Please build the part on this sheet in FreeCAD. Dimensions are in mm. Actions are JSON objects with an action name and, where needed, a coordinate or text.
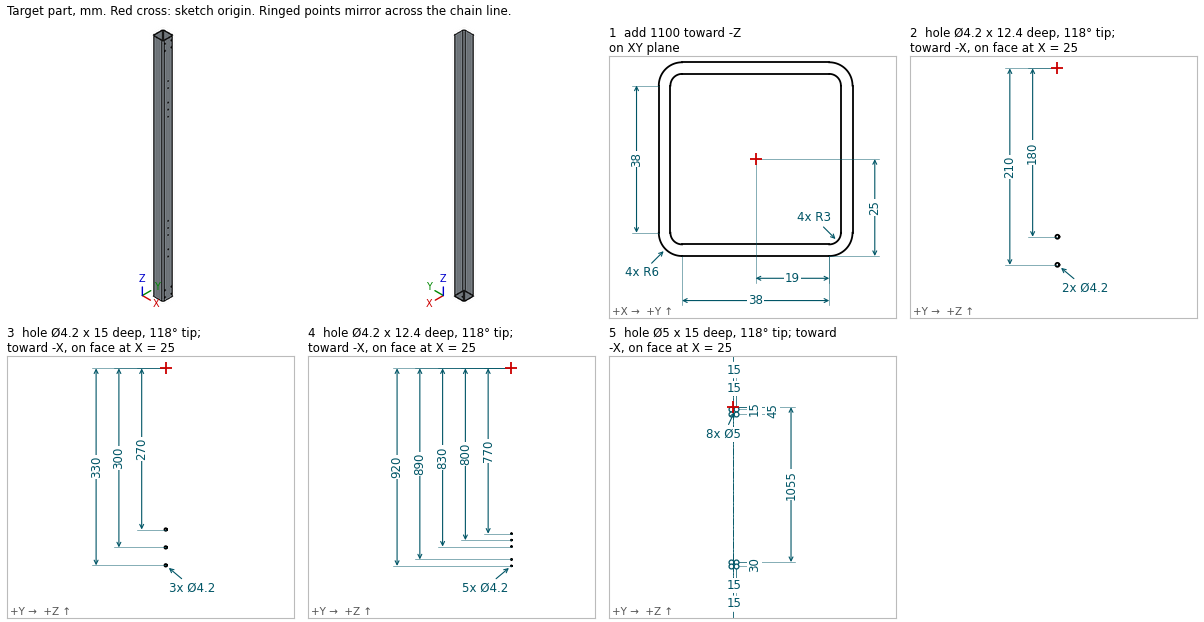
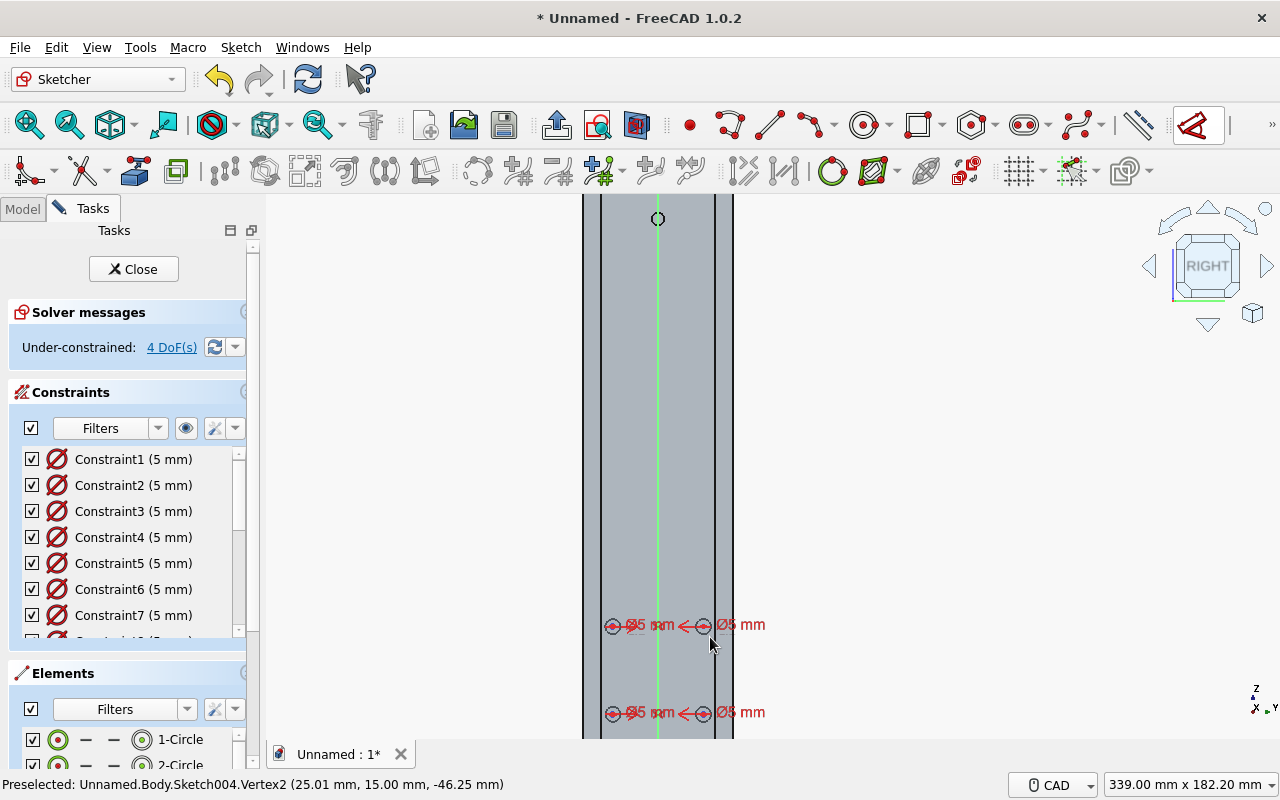
{"action": "left_click", "coordinate": [704, 627]}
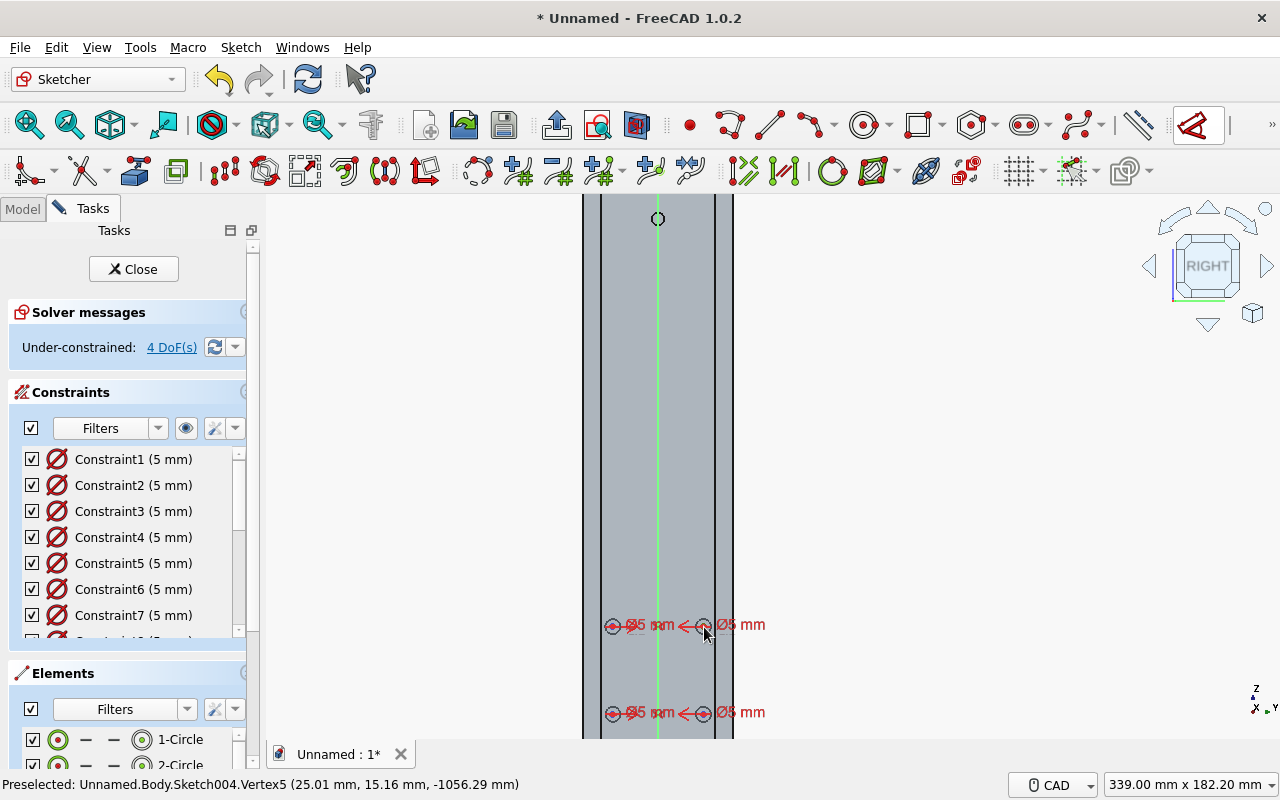
{"action": "key", "text": "l"}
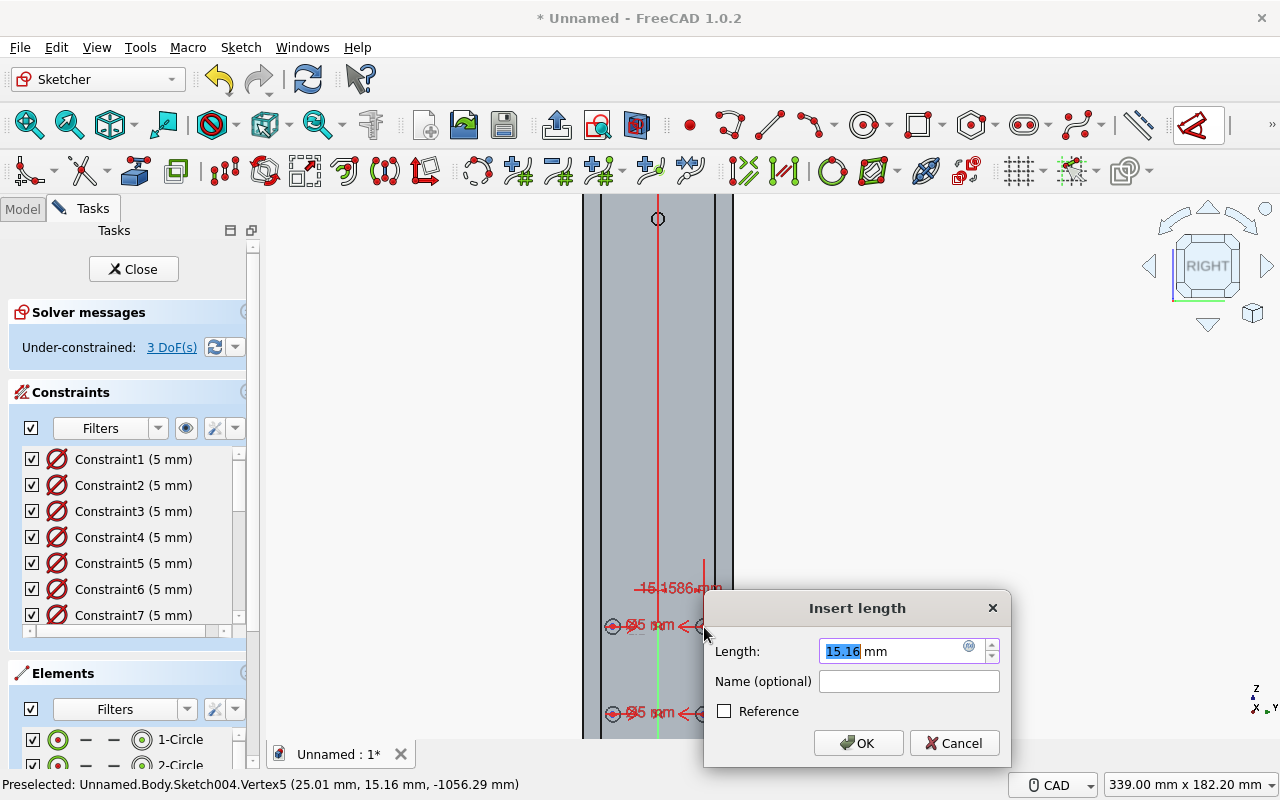
{"action": "type", "text": "15"}
{"action": "key", "text": "Return"}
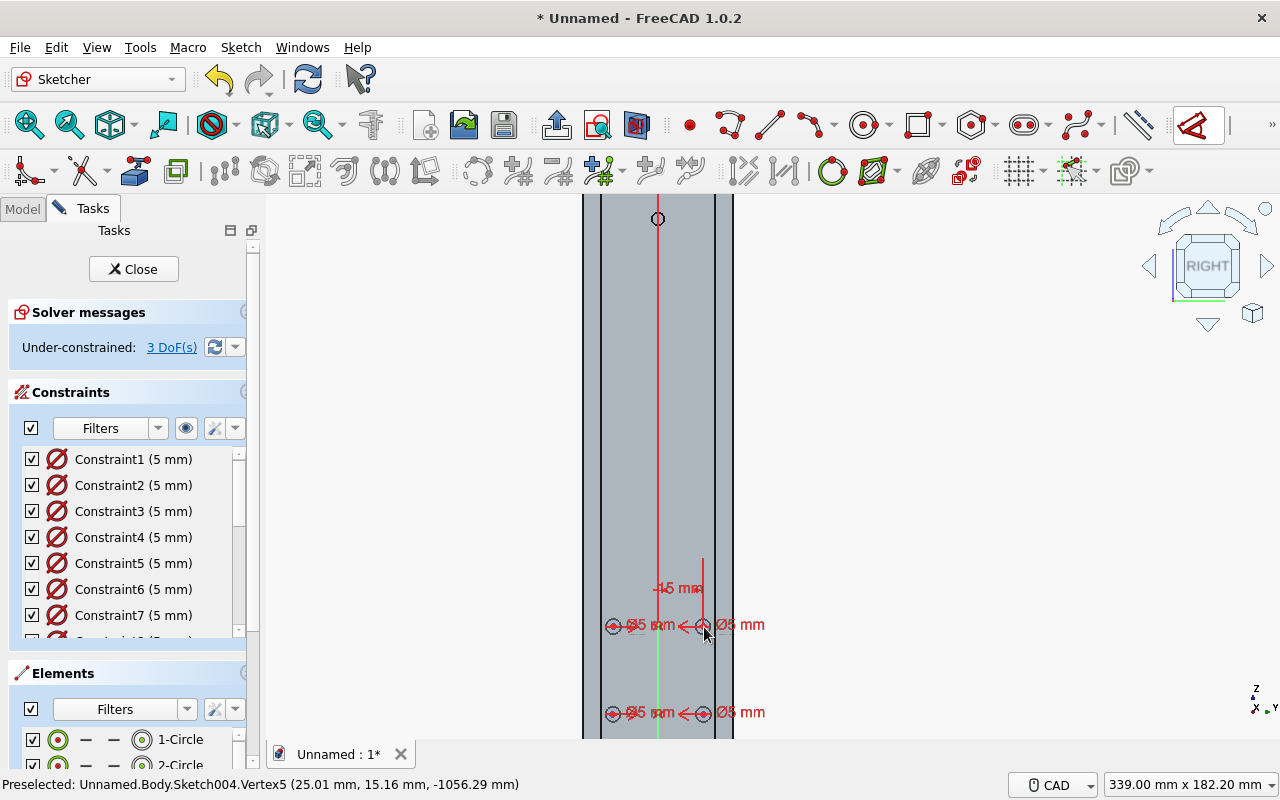
{"action": "scroll", "coordinate": [710, 638], "scroll_direction": "down", "scroll_amount": 11}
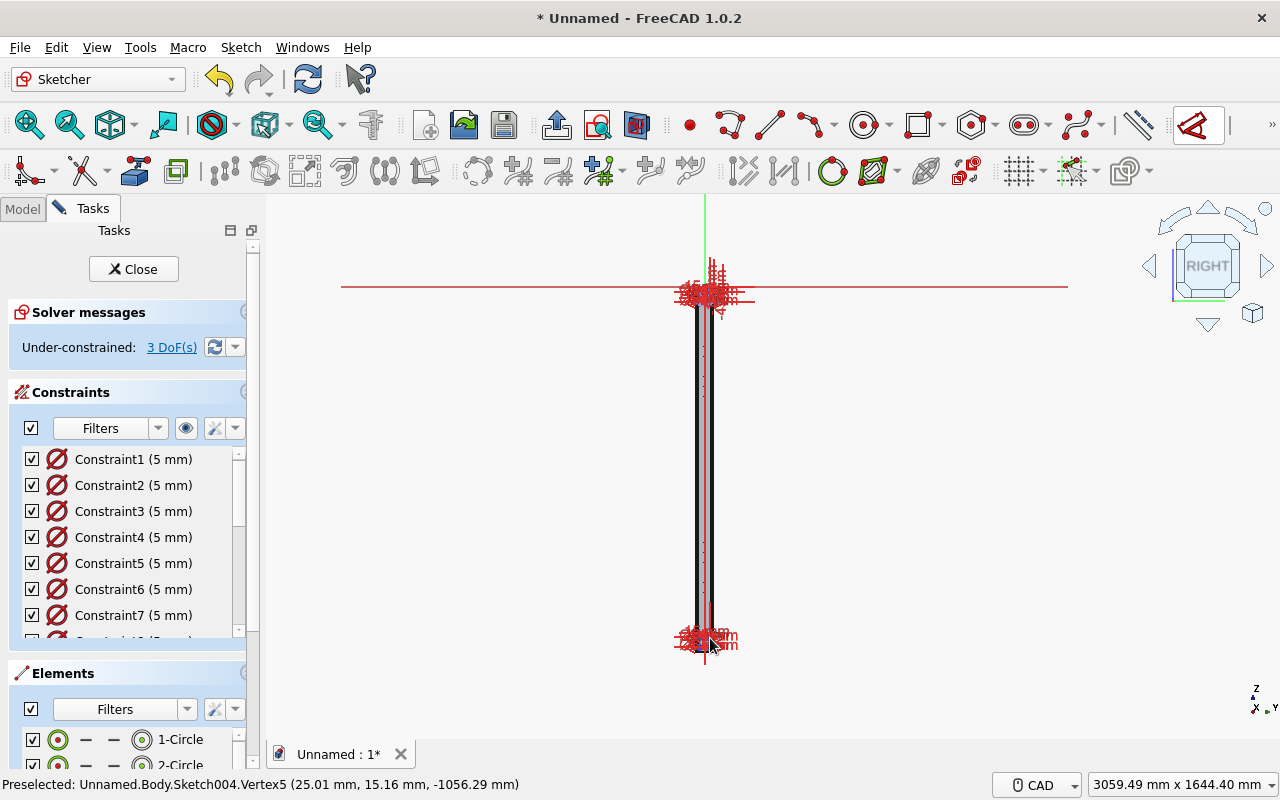
{"action": "scroll", "coordinate": [710, 647], "scroll_direction": "up", "scroll_amount": 11}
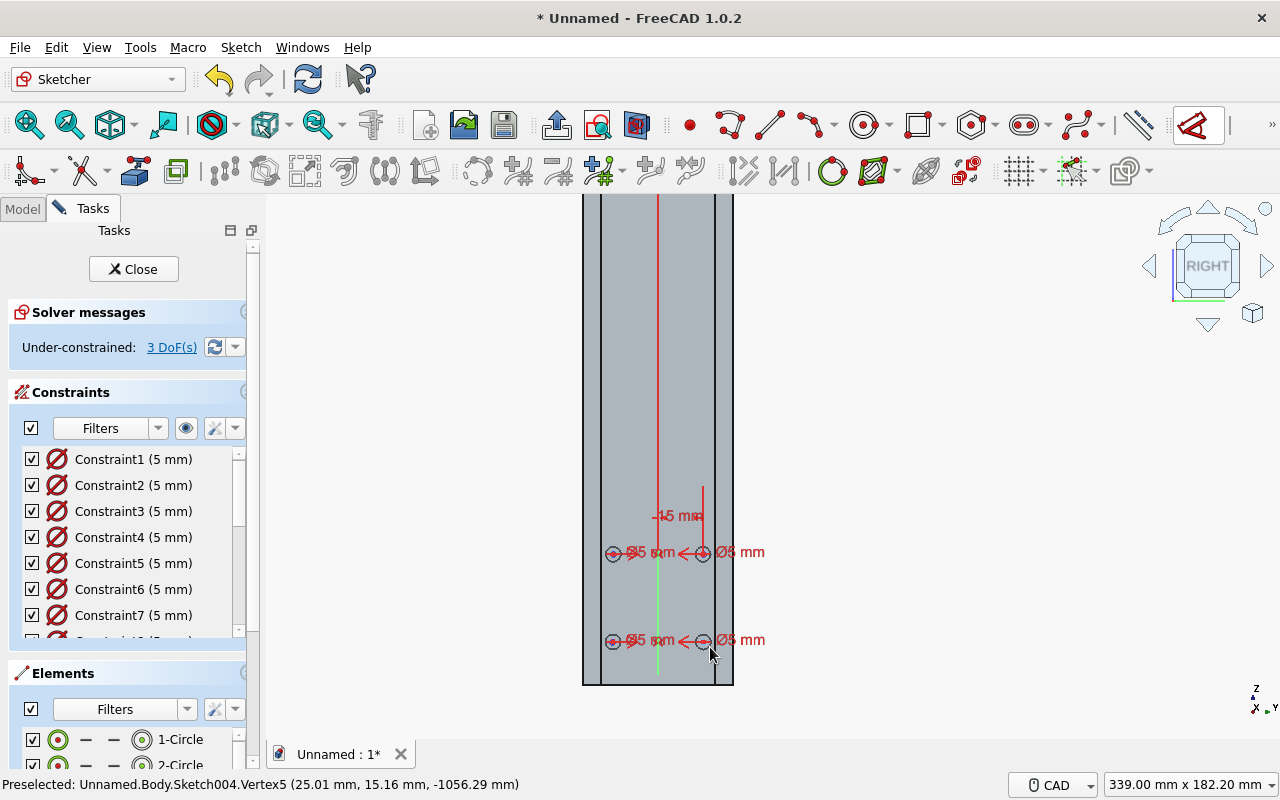
{"action": "left_click", "coordinate": [703, 642]}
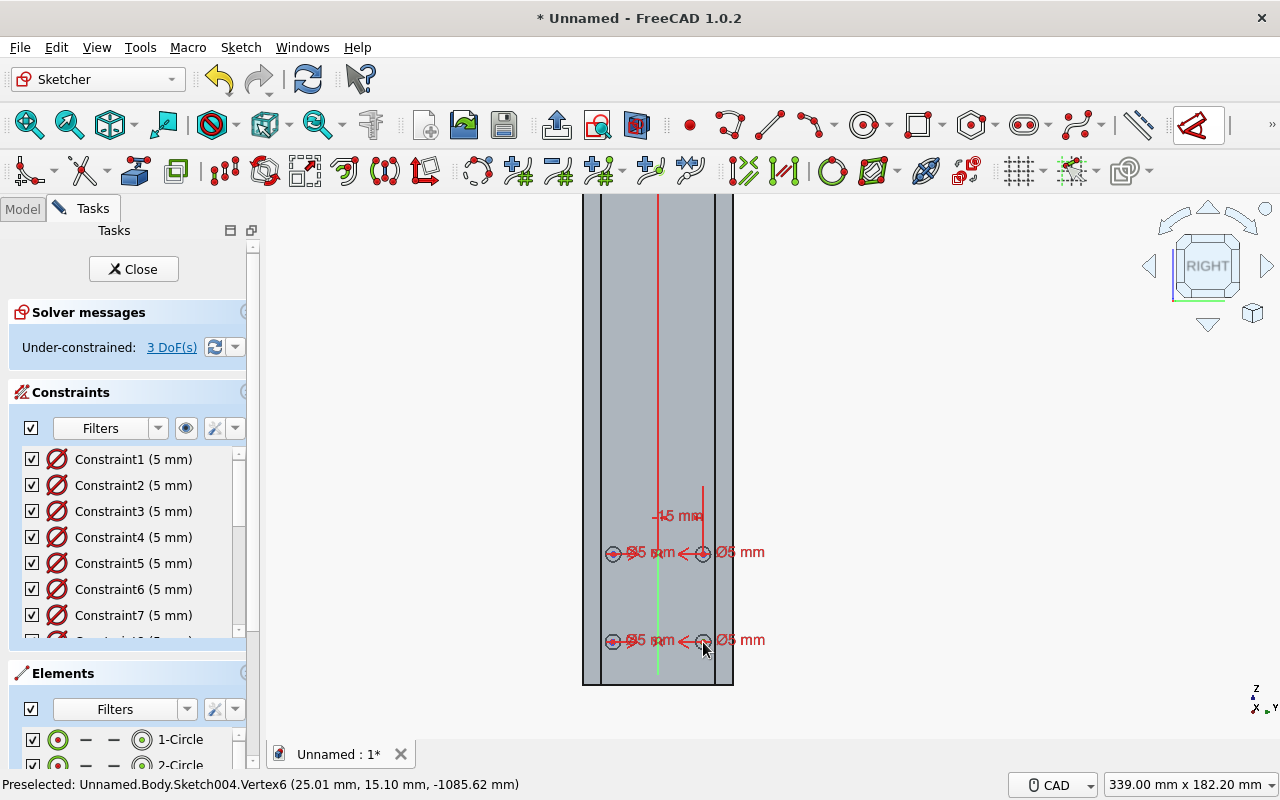
{"action": "left_click", "coordinate": [1218, 126]}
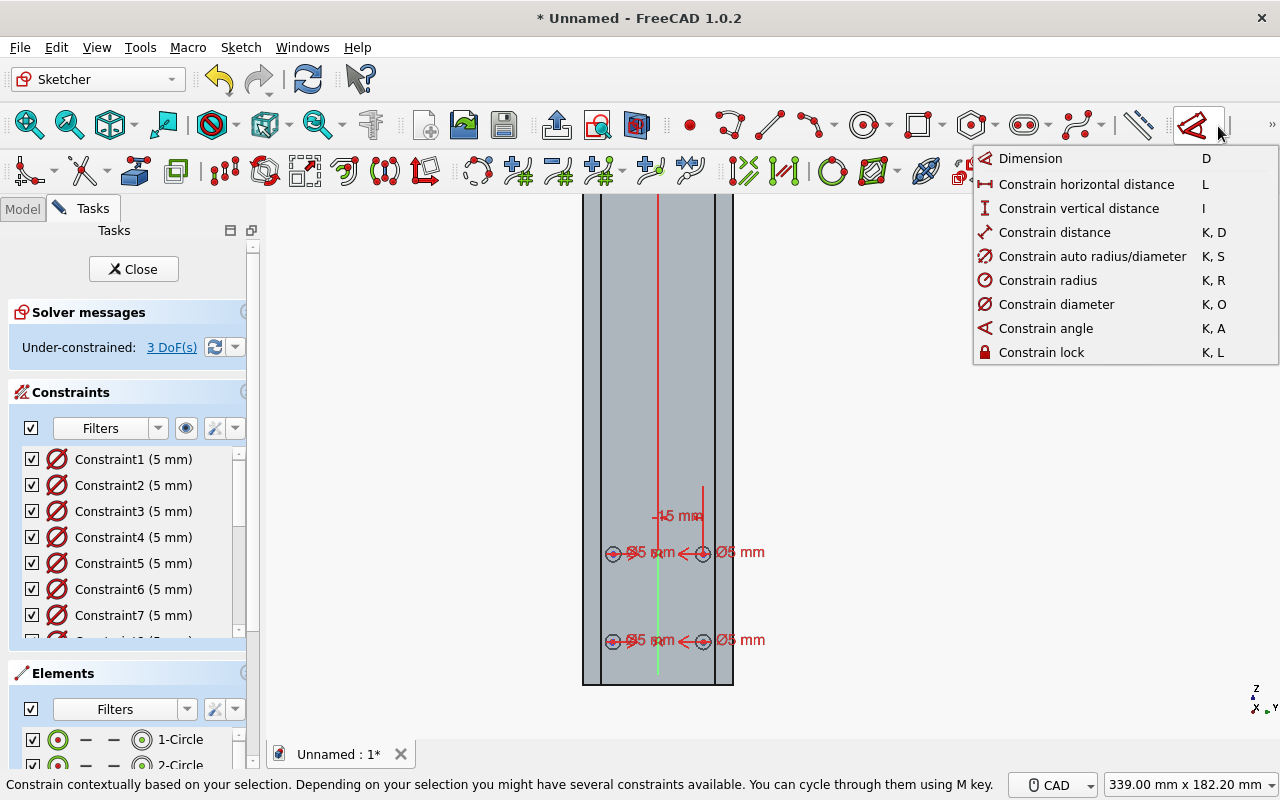
{"action": "left_click", "coordinate": [1126, 184]}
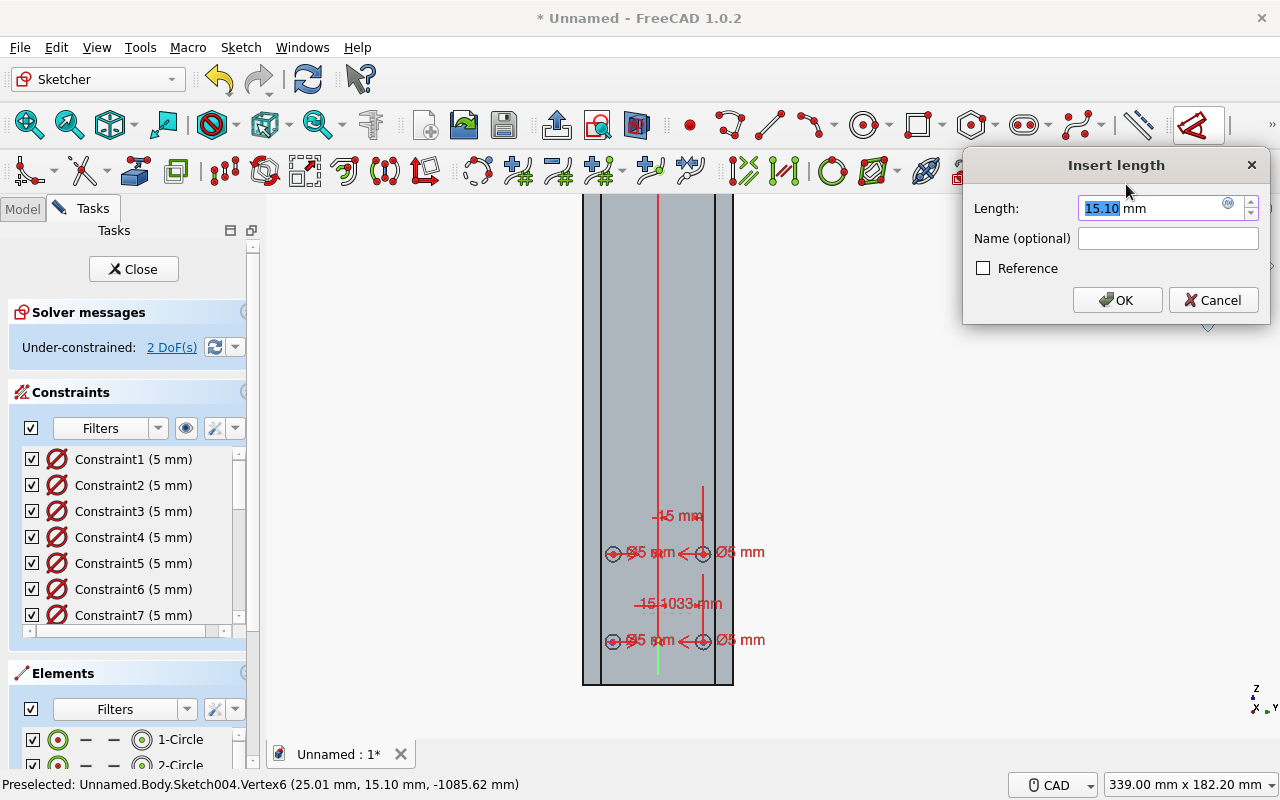
{"action": "type", "text": "15"}
{"action": "key", "text": "Return"}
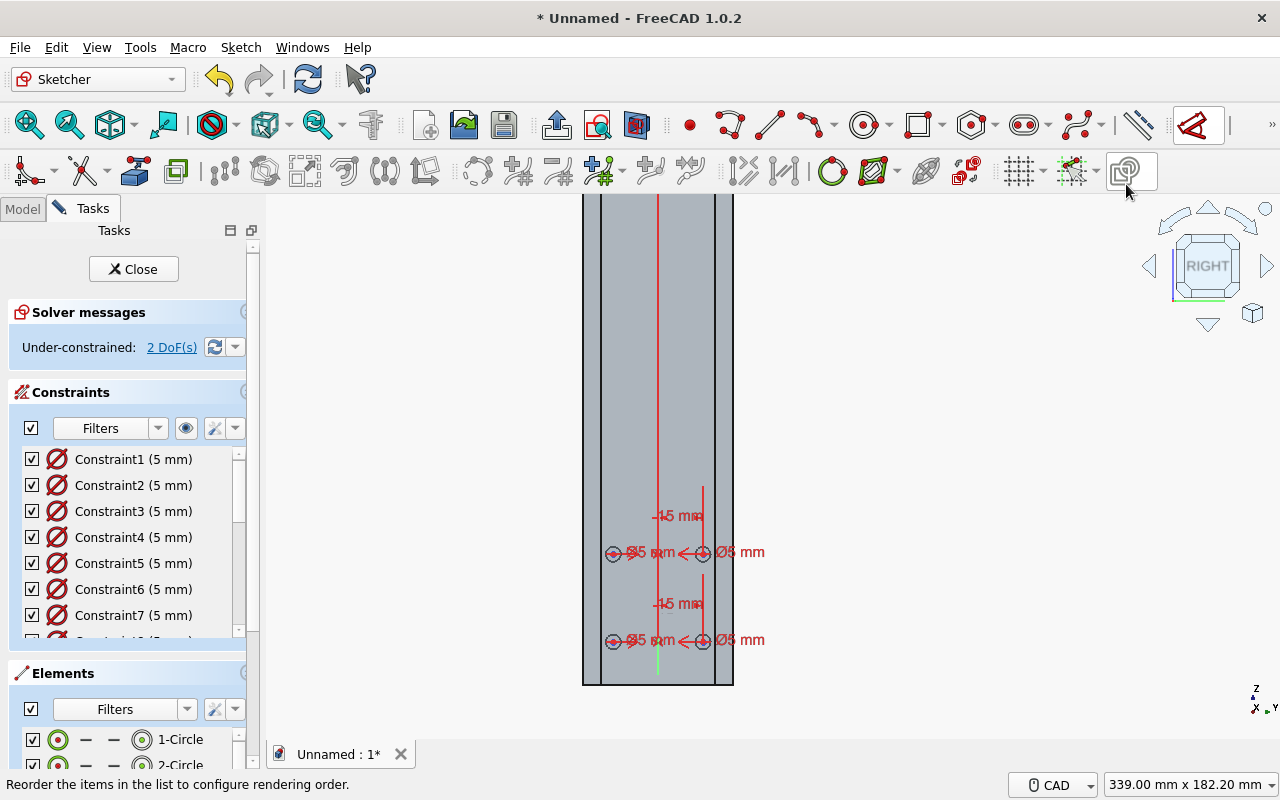
{"action": "left_click", "coordinate": [703, 554]}